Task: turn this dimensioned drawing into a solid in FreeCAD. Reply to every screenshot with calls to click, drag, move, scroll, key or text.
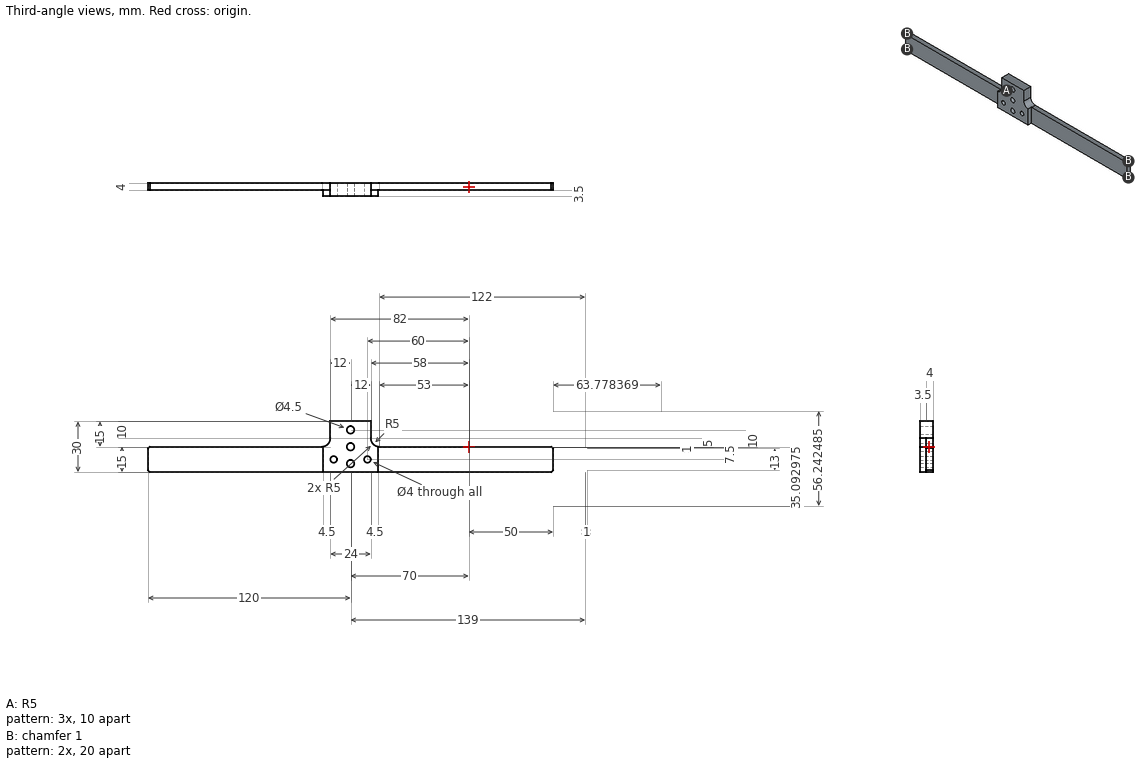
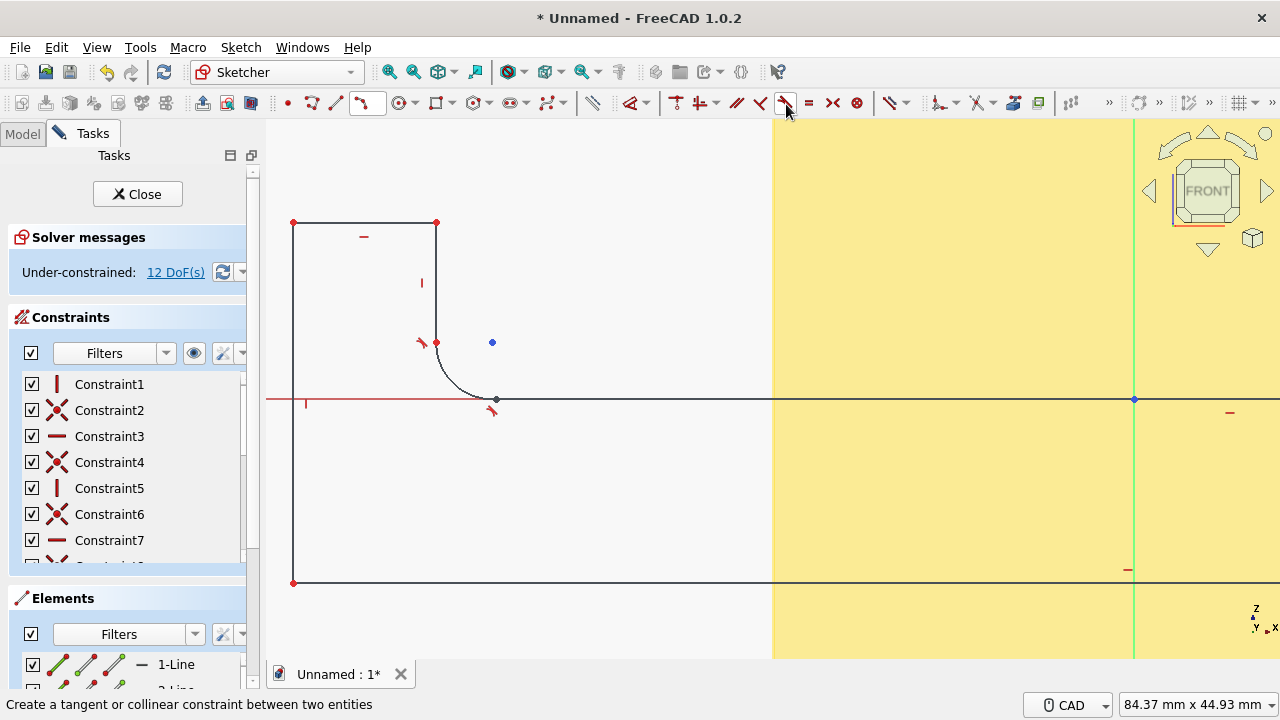
click(443, 370)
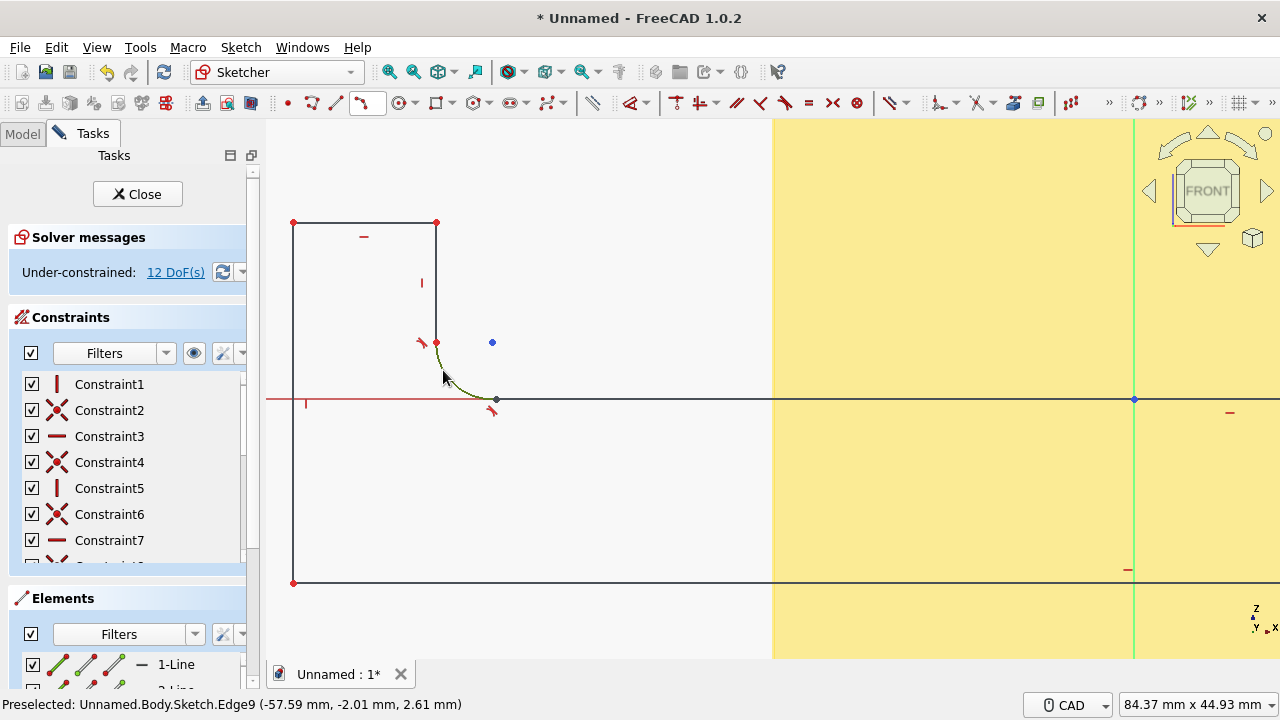
click(648, 104)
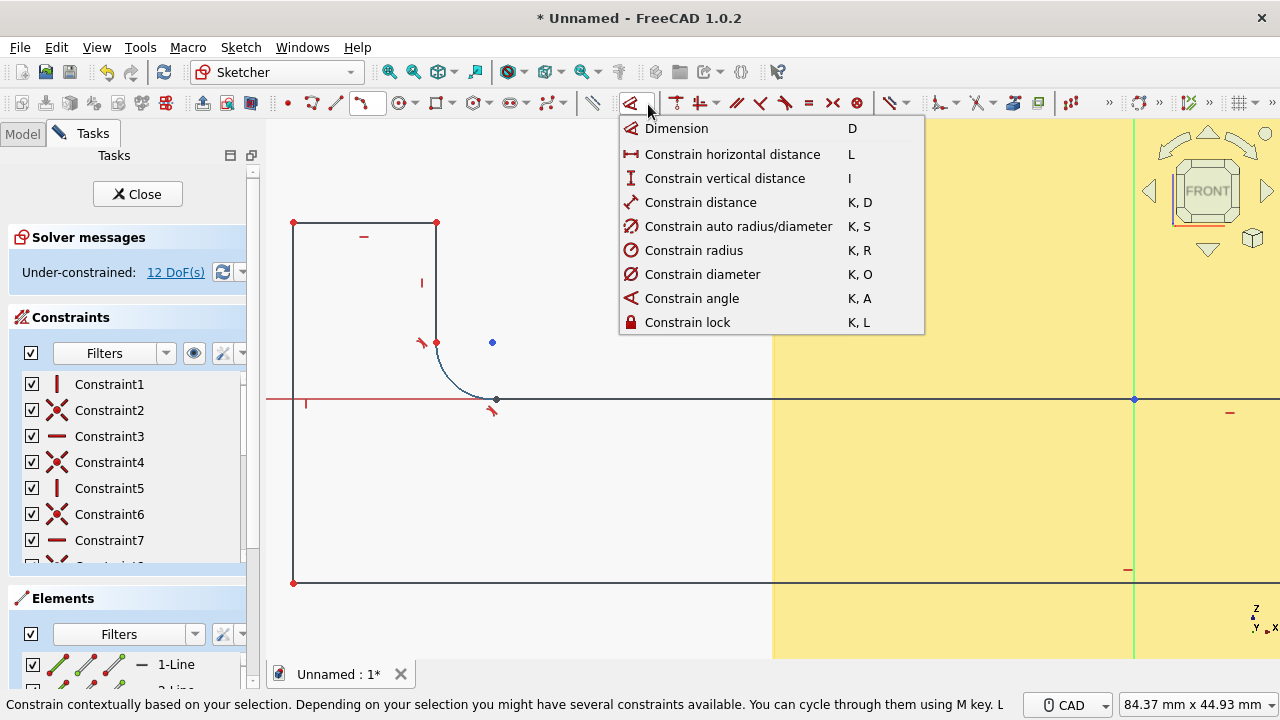
click(772, 250)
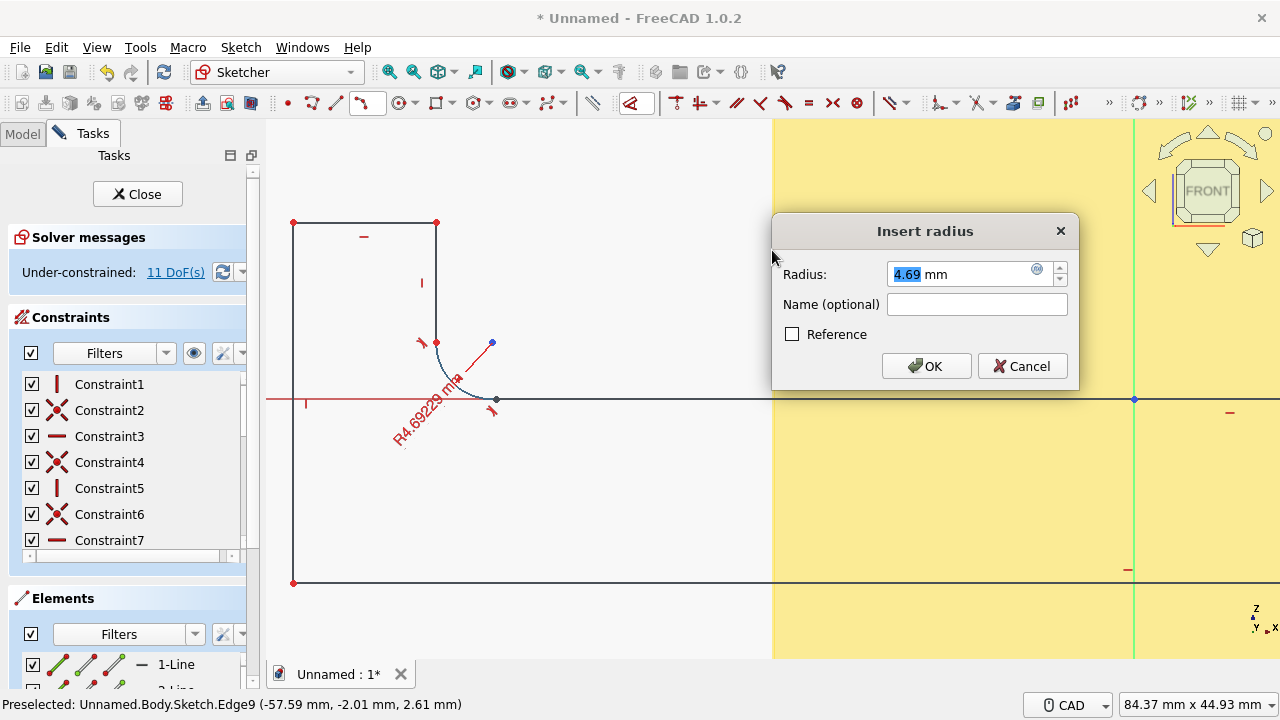
text(5)
key(Return)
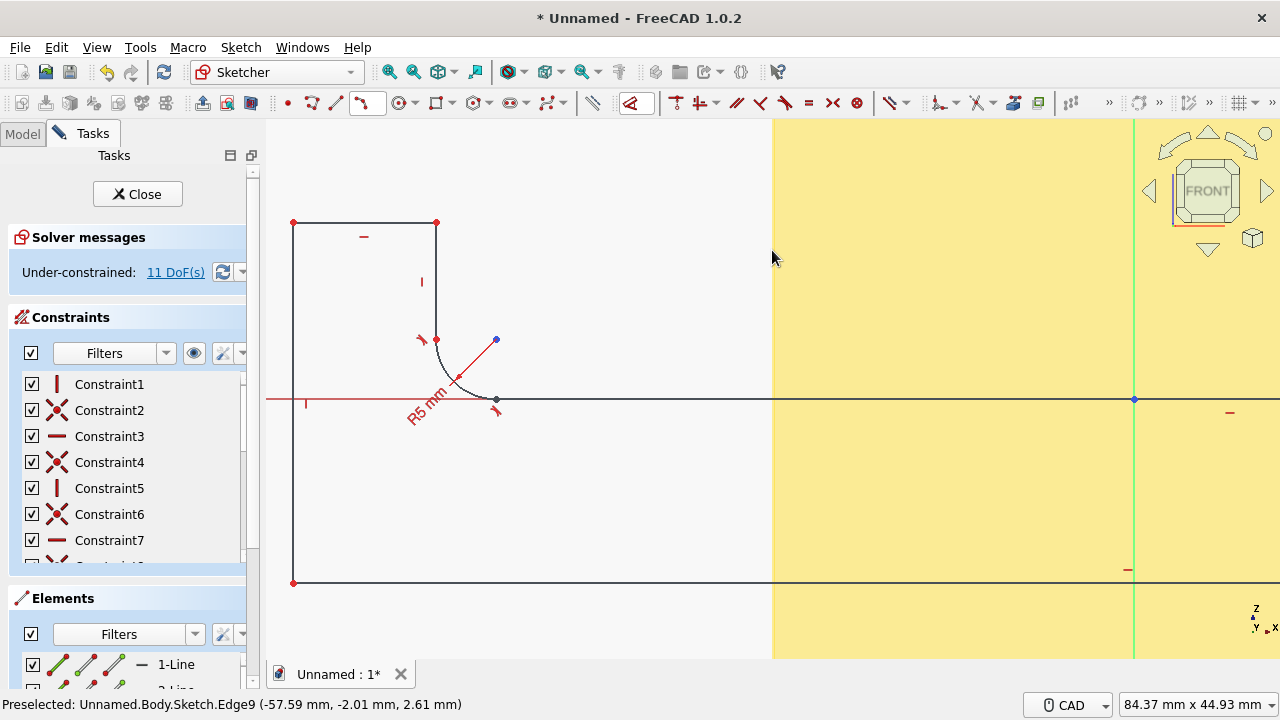
click(436, 304)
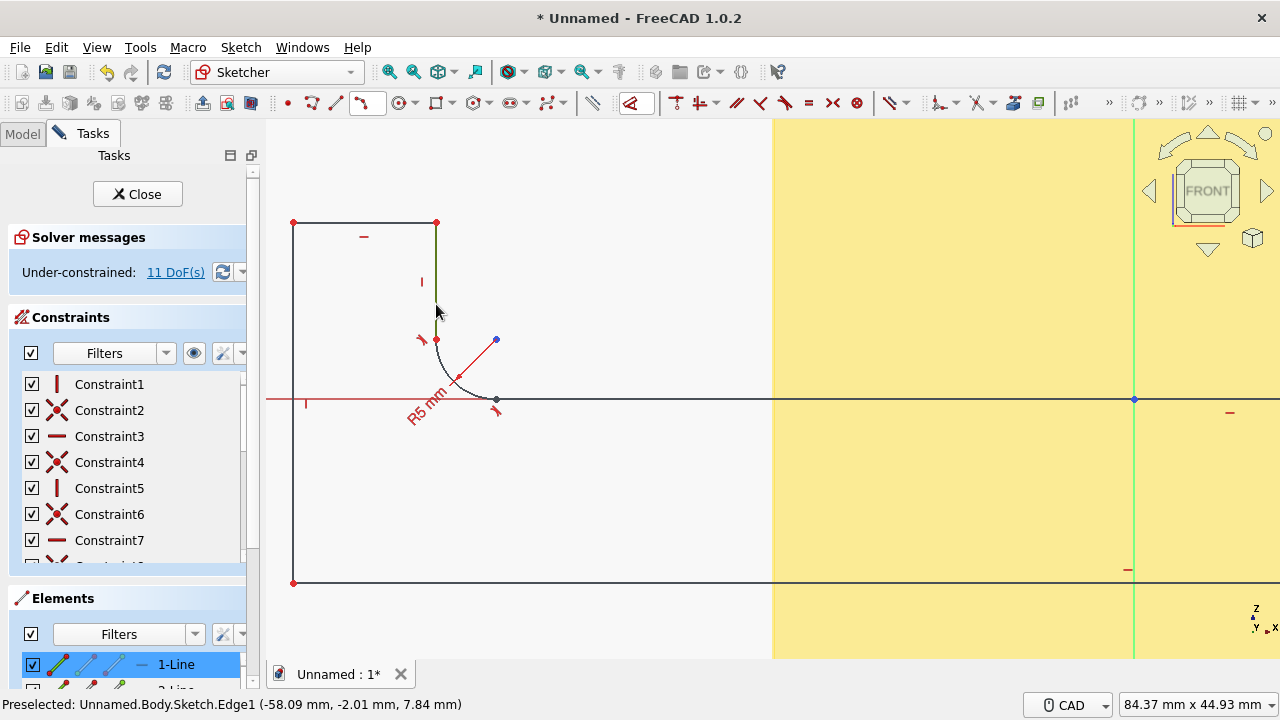
click(648, 104)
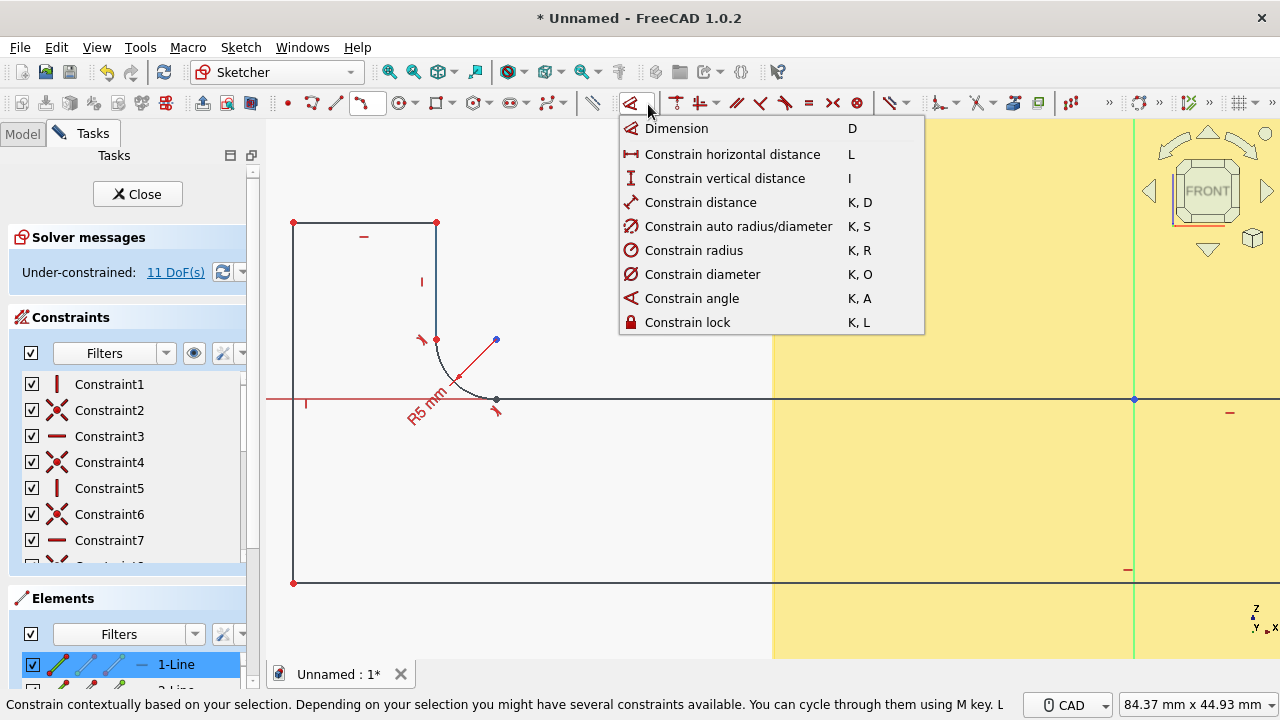
click(772, 178)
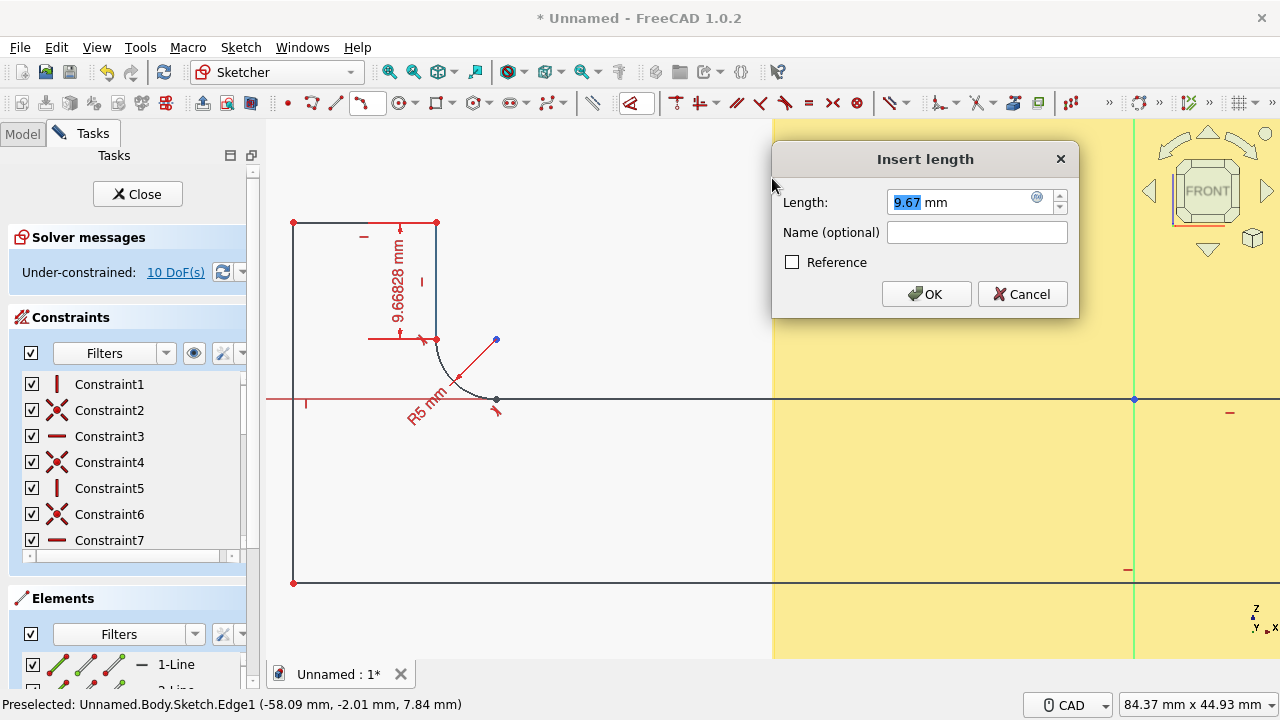
text(10)
key(Return)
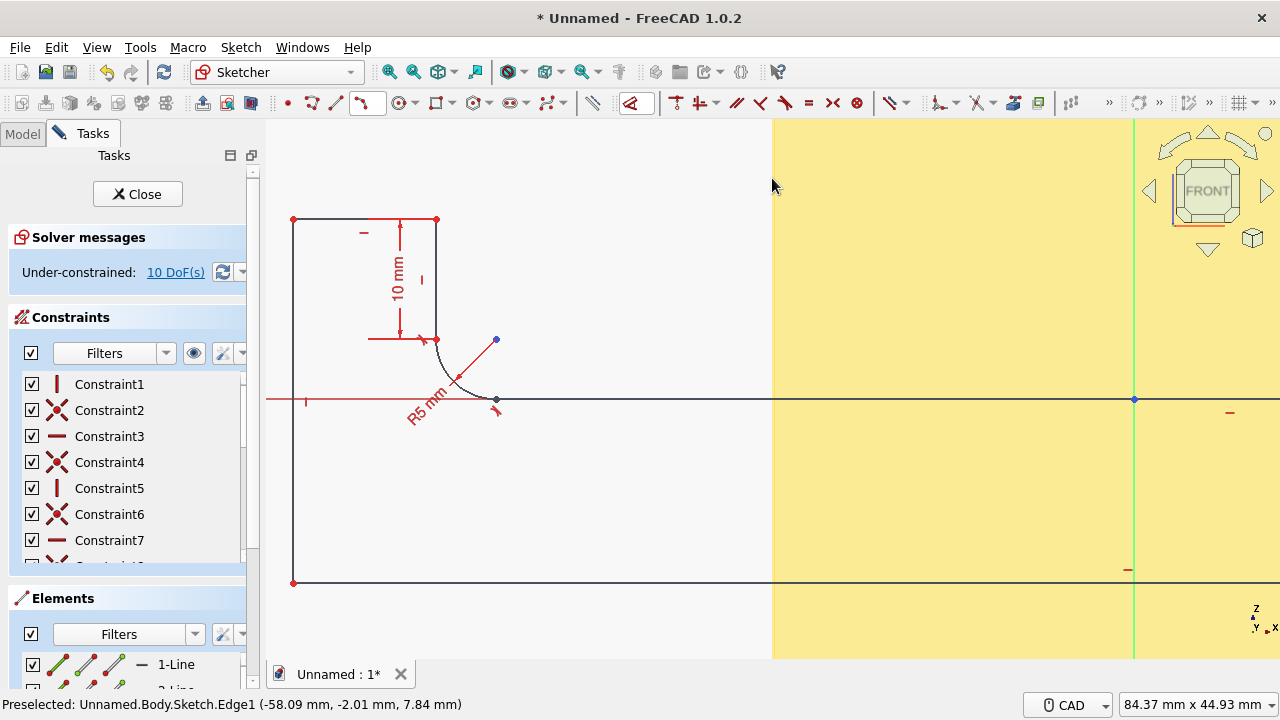
click(393, 219)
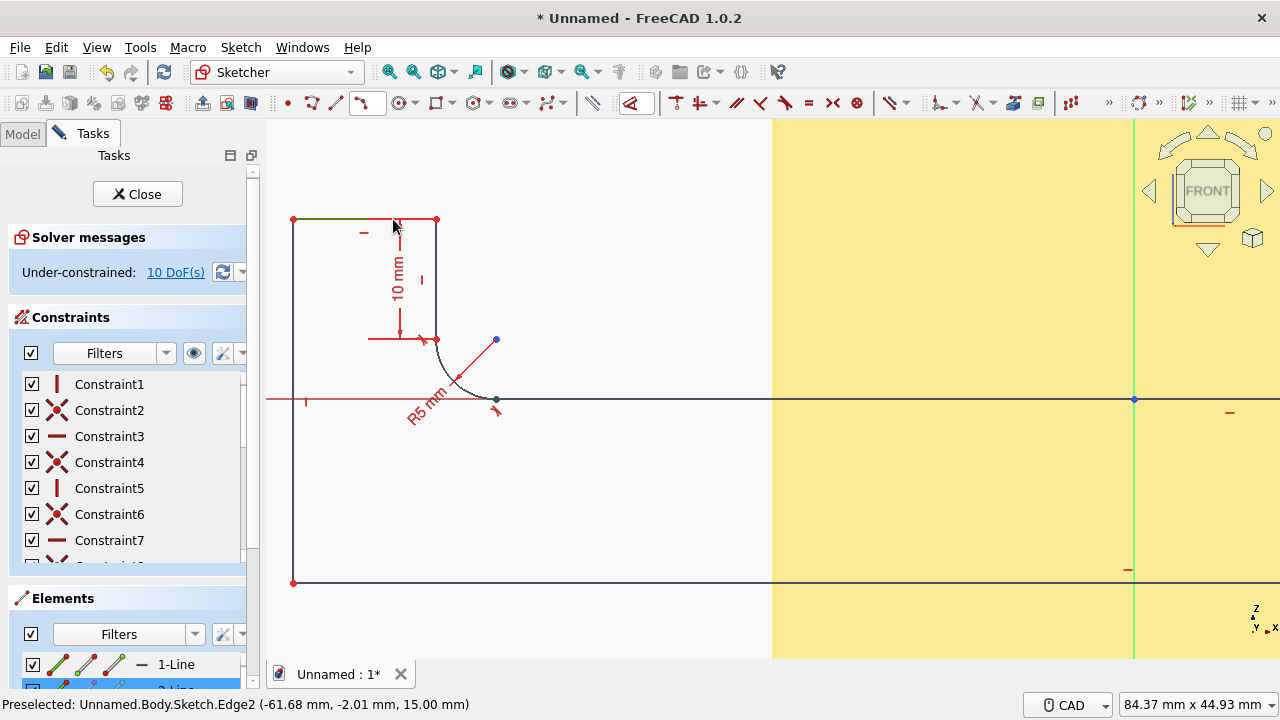
key(l)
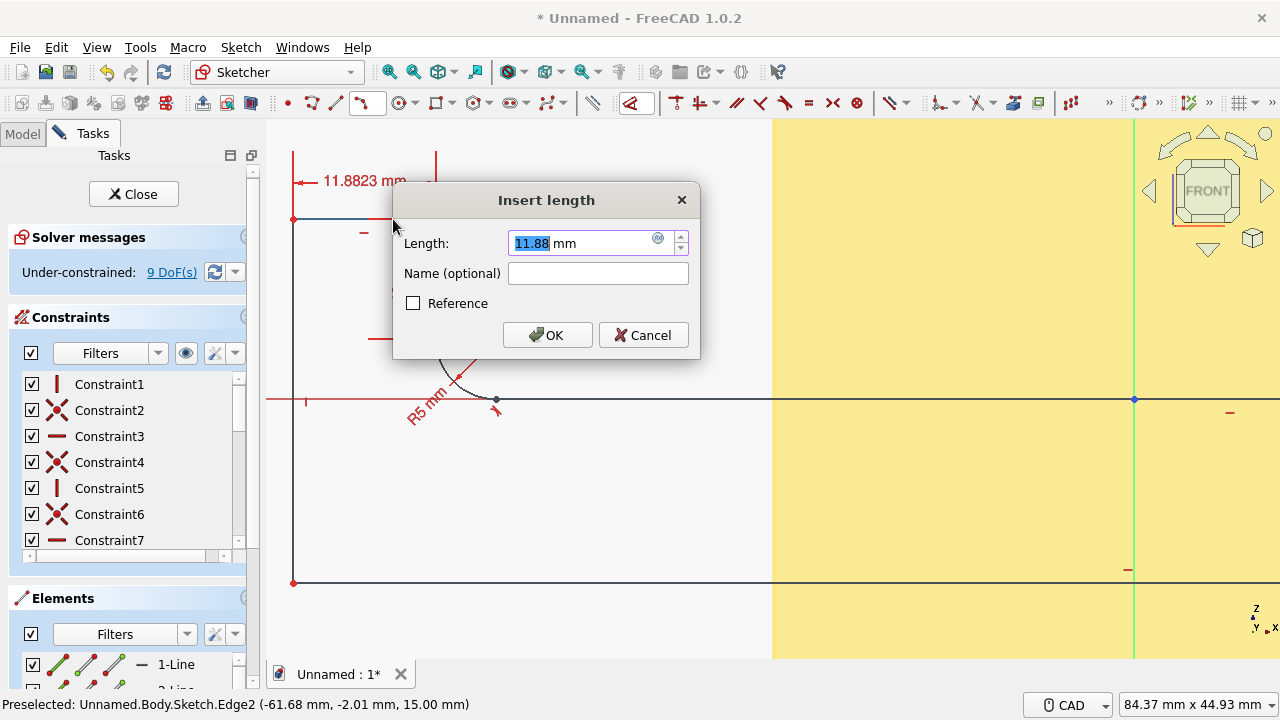
text(12)
key(Return)